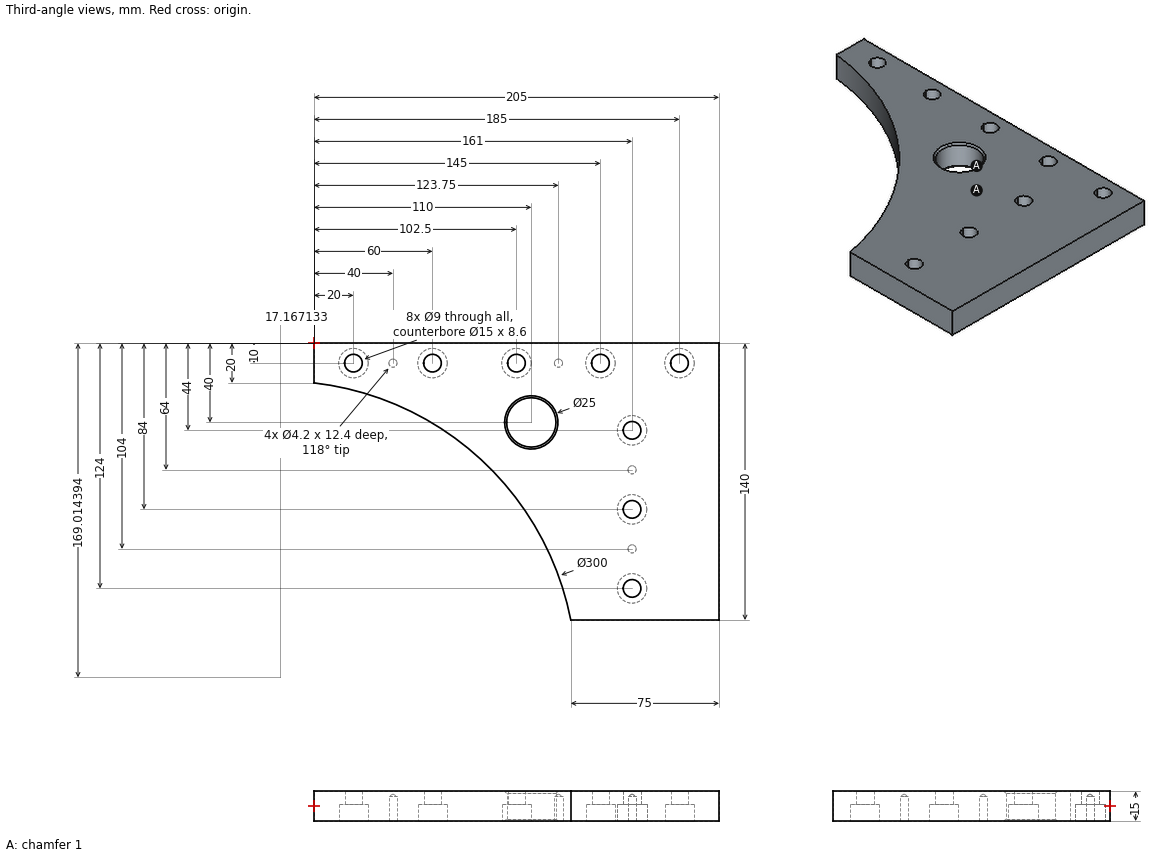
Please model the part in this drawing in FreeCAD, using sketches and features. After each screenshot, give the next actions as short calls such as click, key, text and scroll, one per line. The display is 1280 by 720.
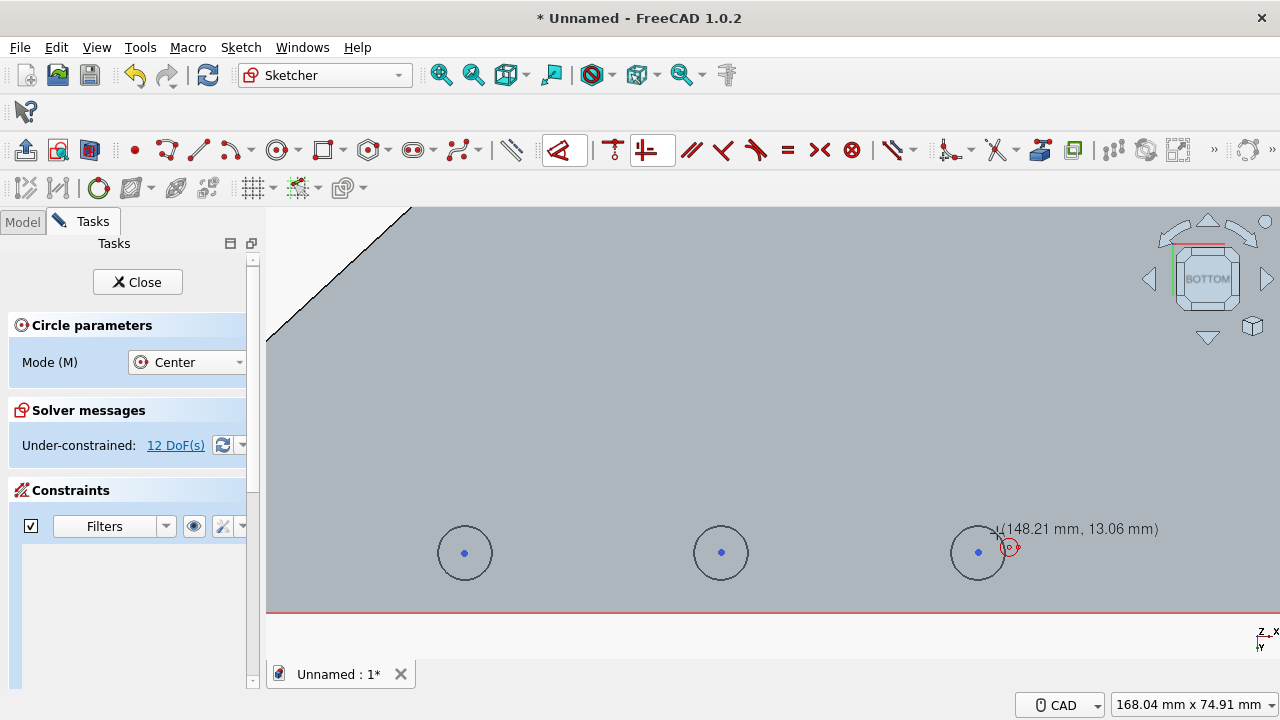
click(1074, 347)
click(1093, 328)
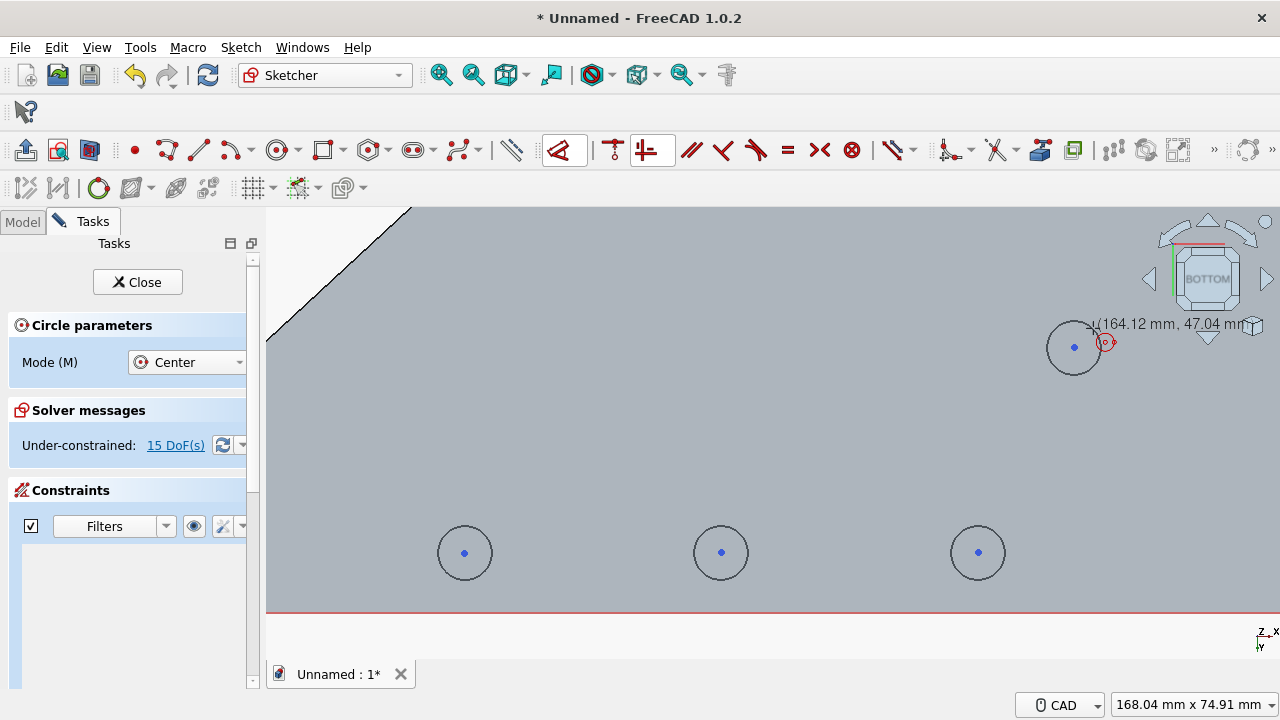
scroll(722, 554, down, 5)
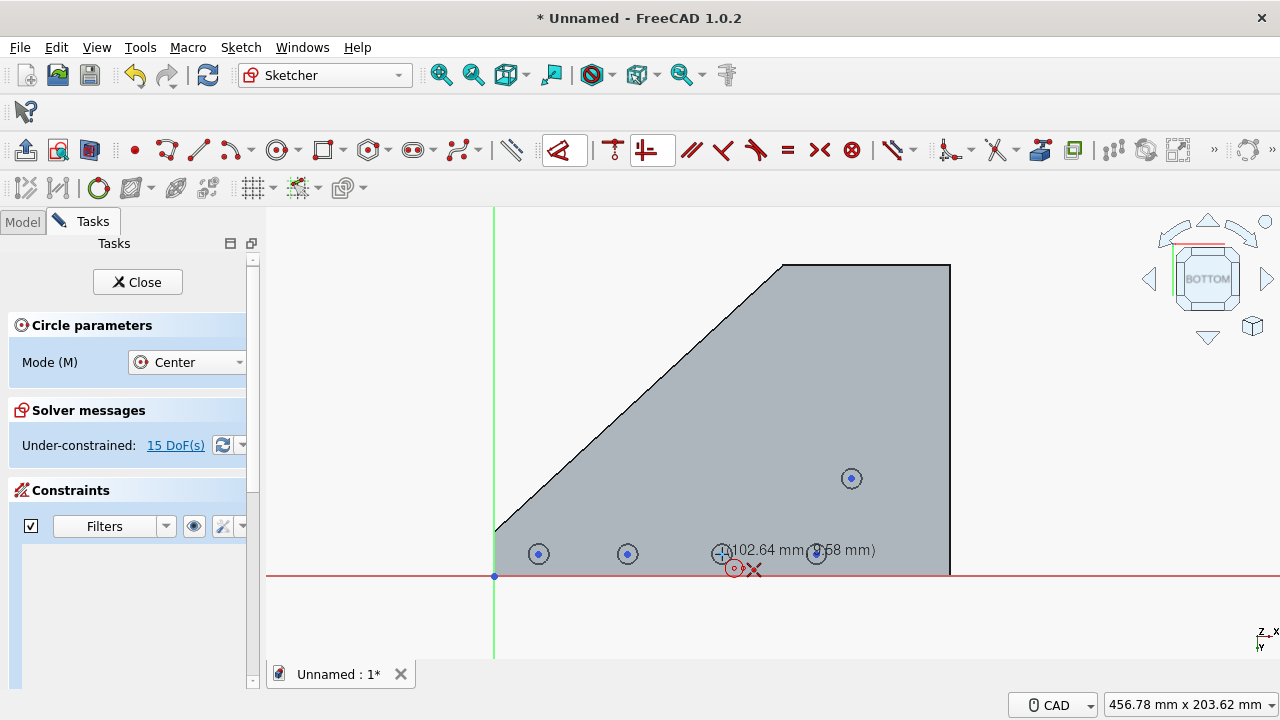
scroll(852, 390, up, 5)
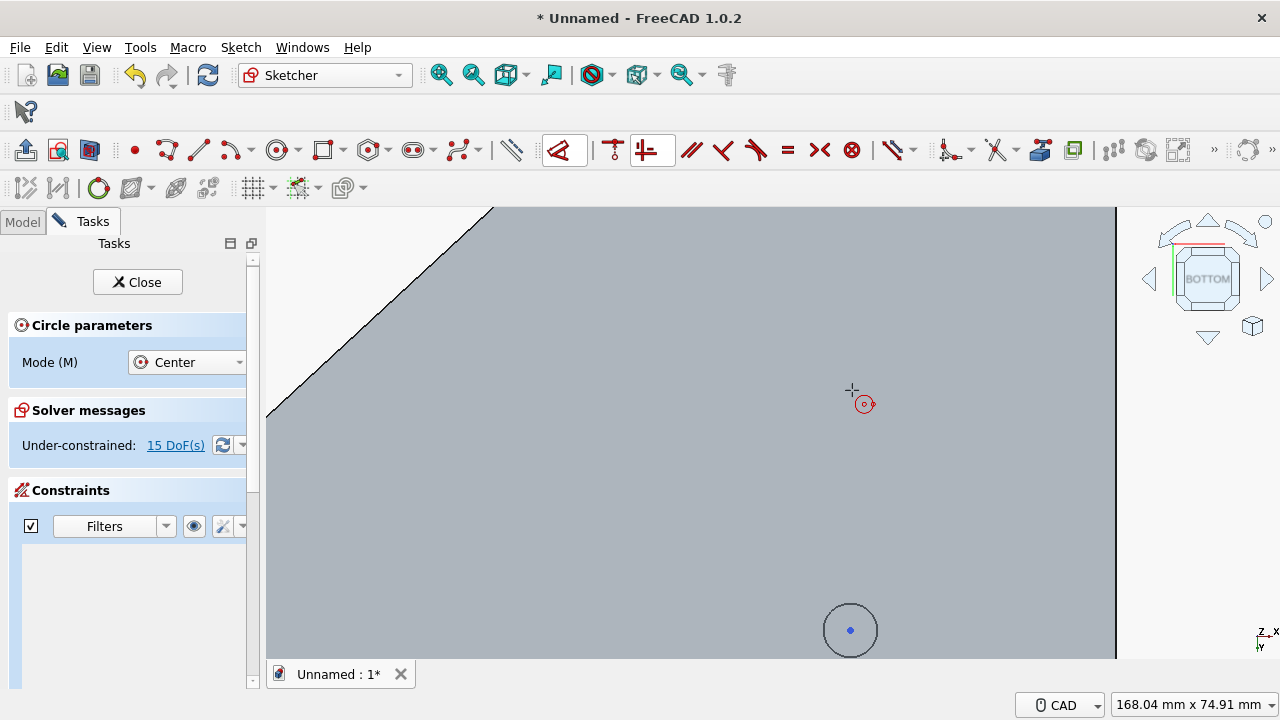
click(851, 388)
click(870, 369)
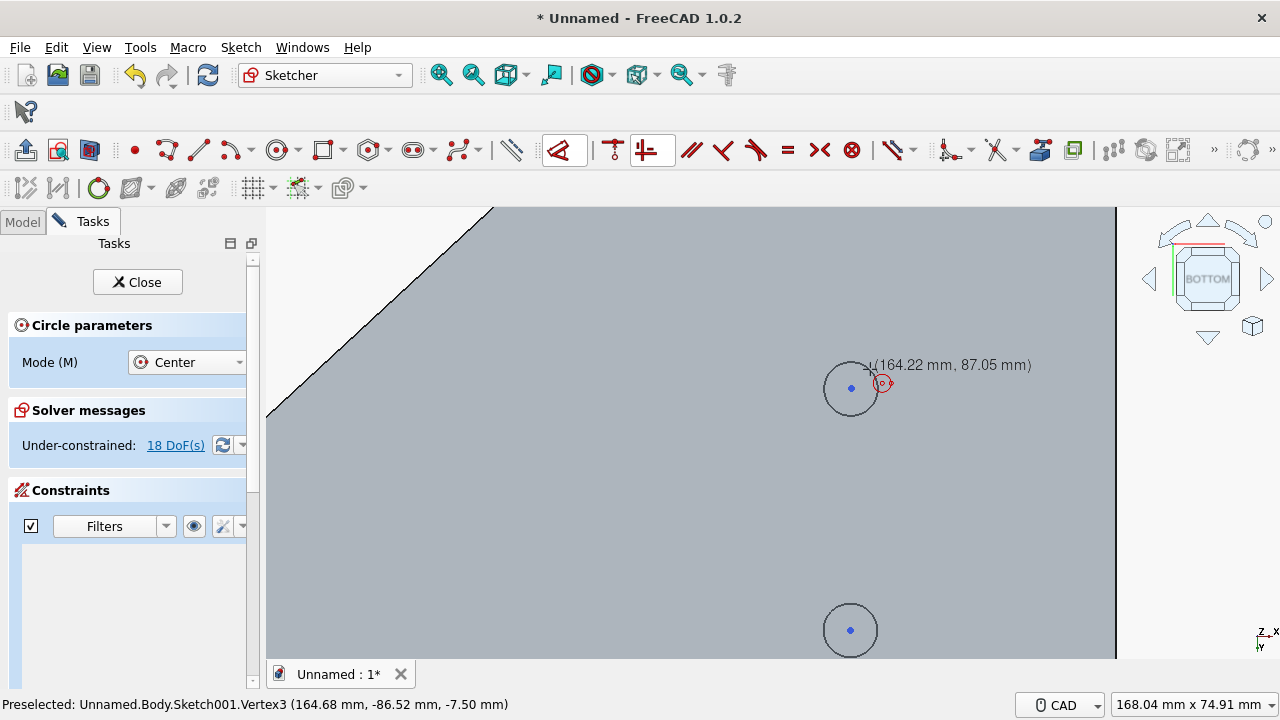
scroll(852, 390, down, 5)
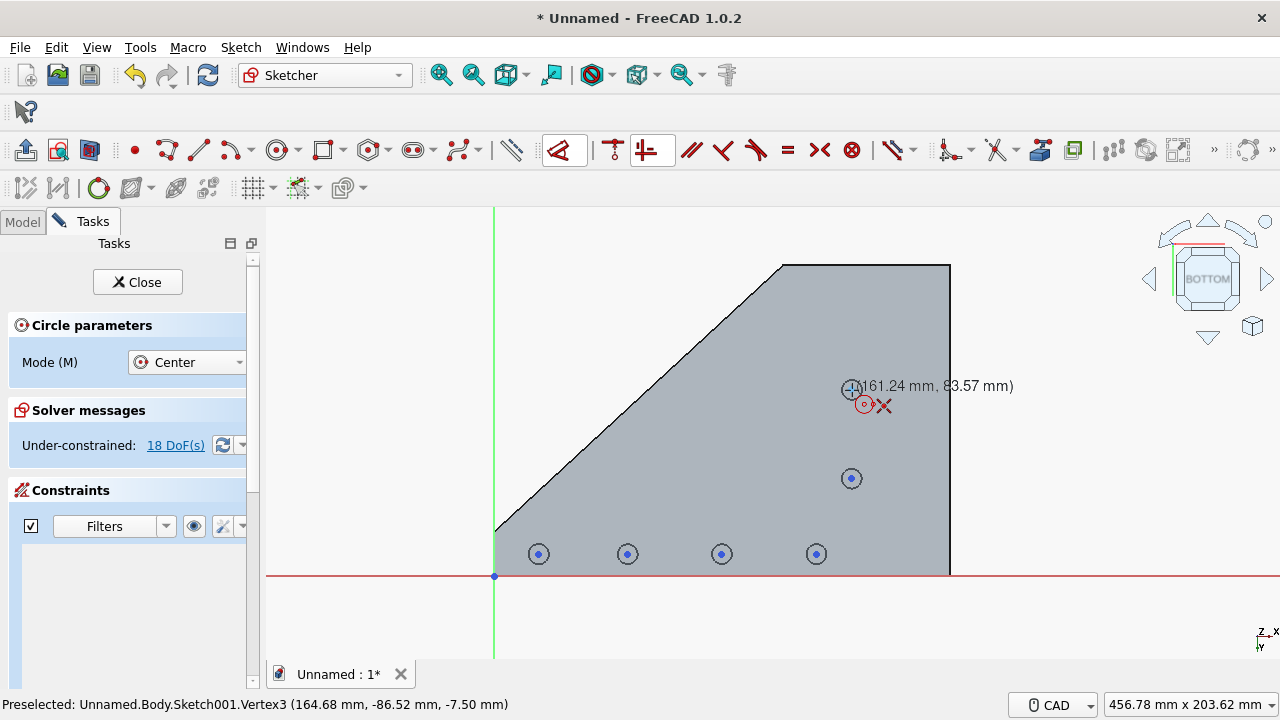
scroll(852, 301, up, 5)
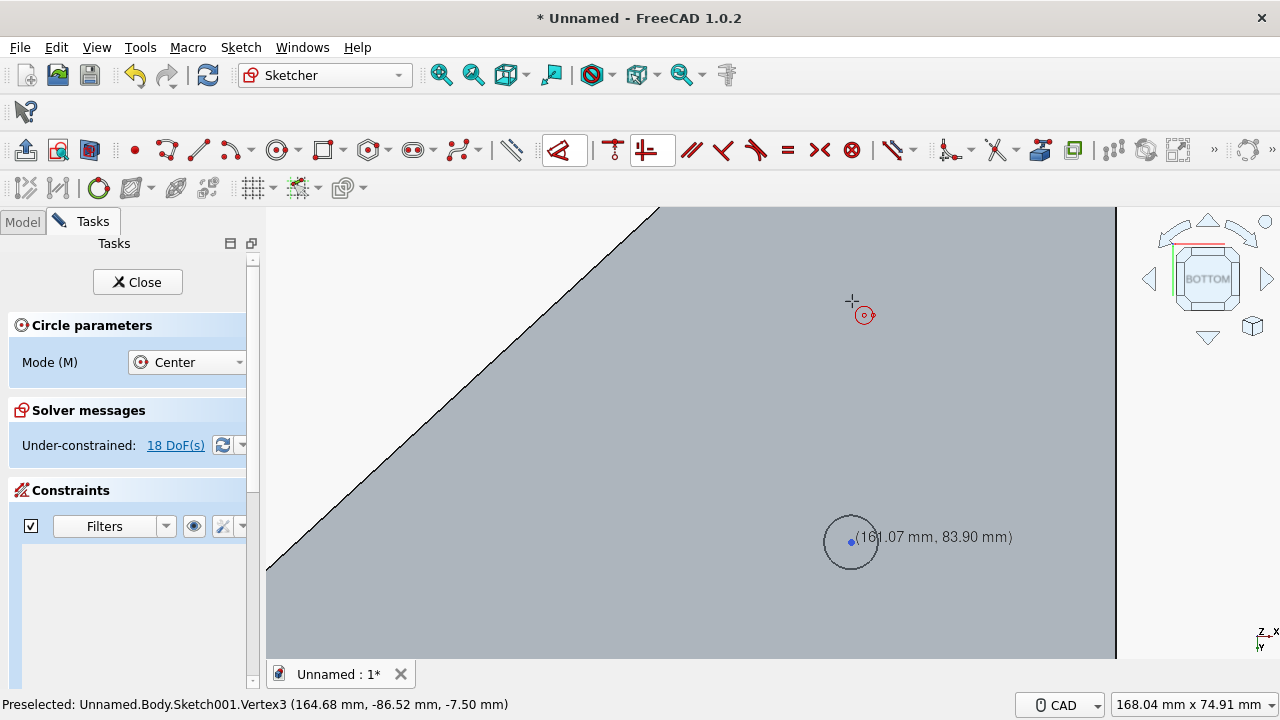
click(851, 300)
click(870, 281)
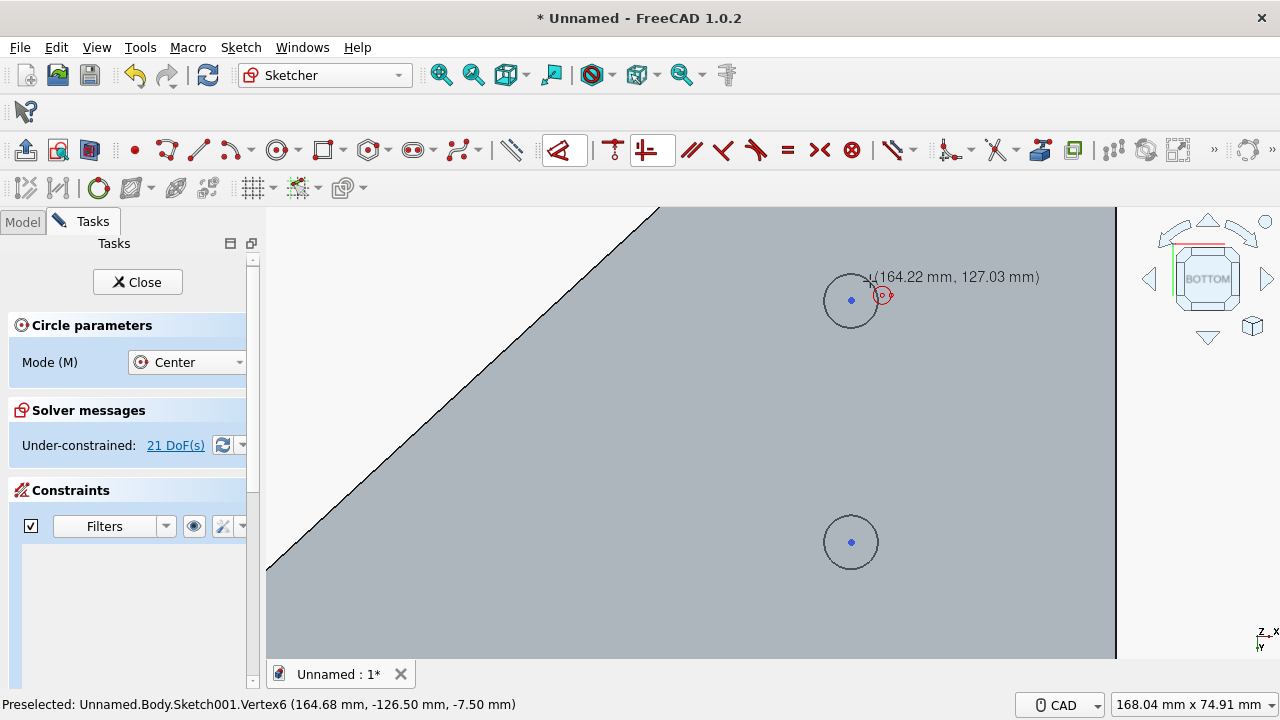
scroll(852, 300, down, 5)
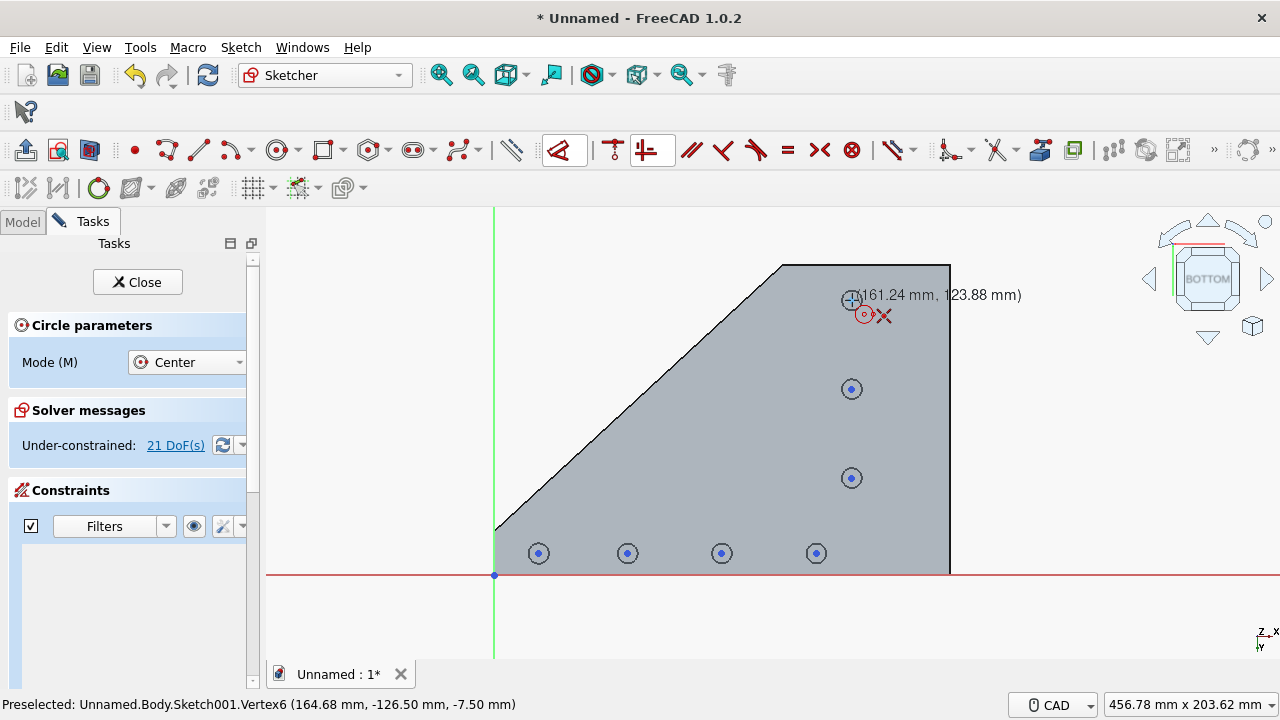
scroll(905, 553, up, 5)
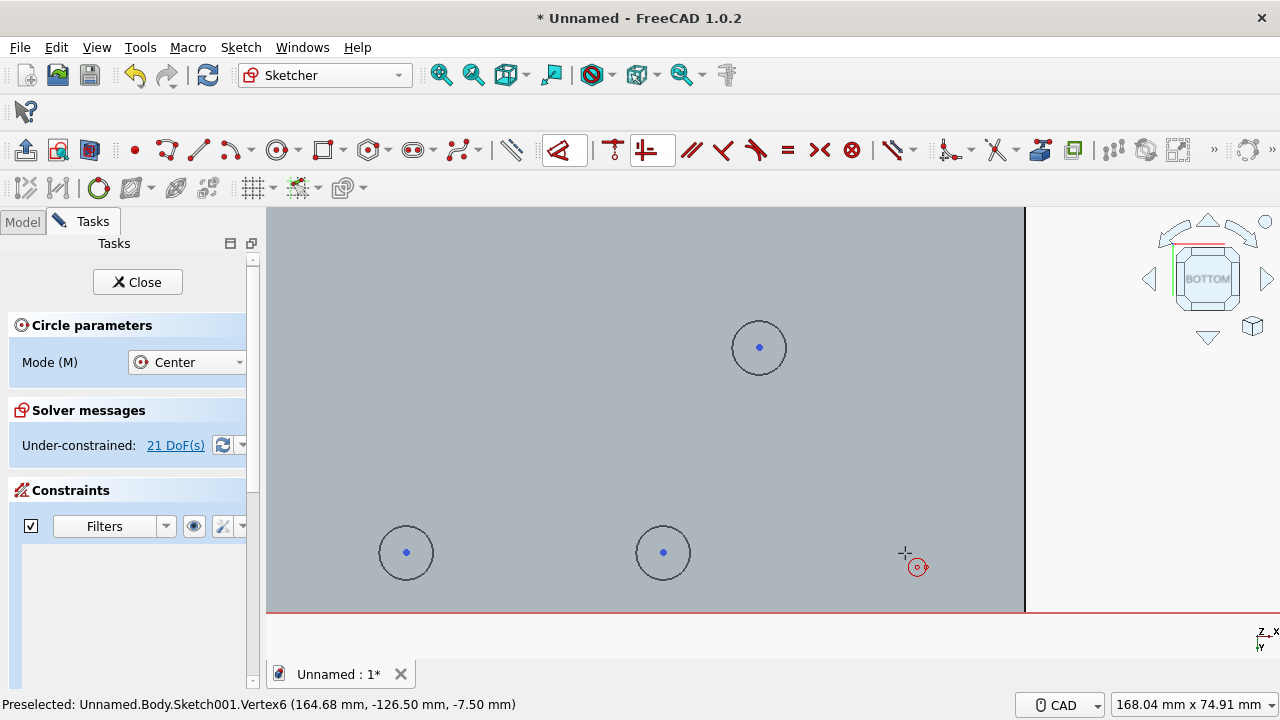
click(904, 552)
click(923, 533)
key(Escape)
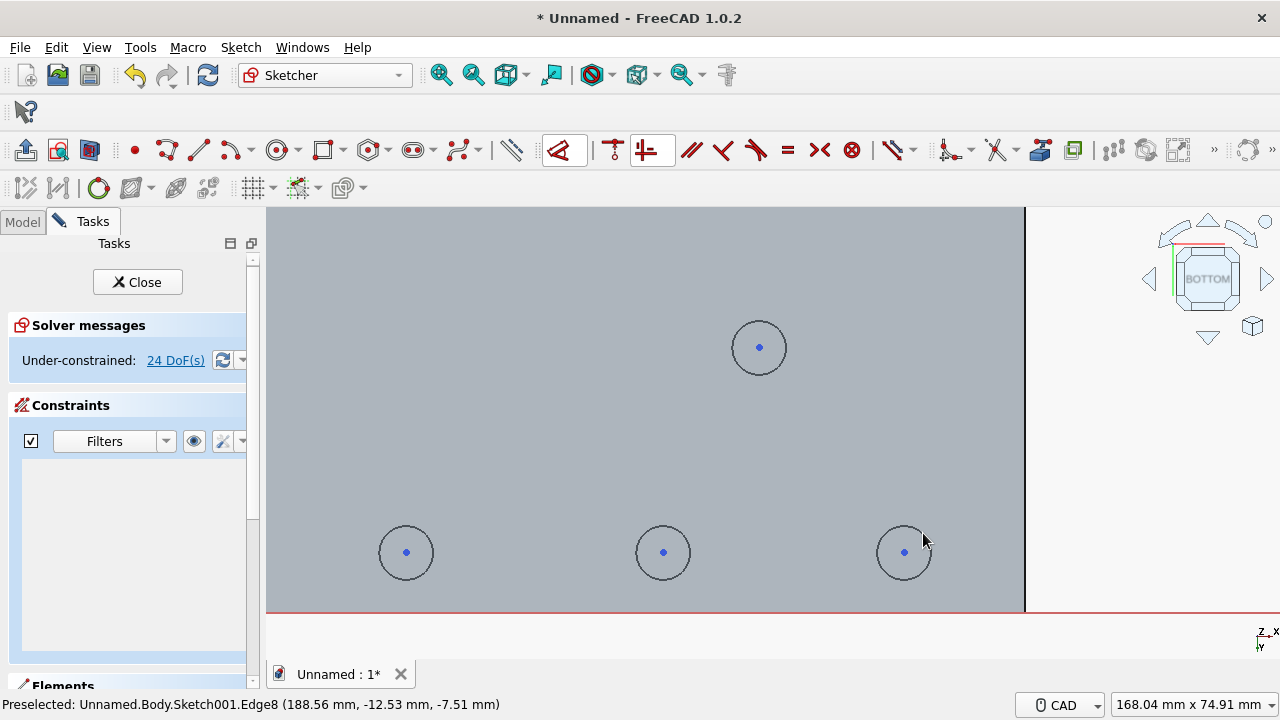
scroll(905, 554, down, 5)